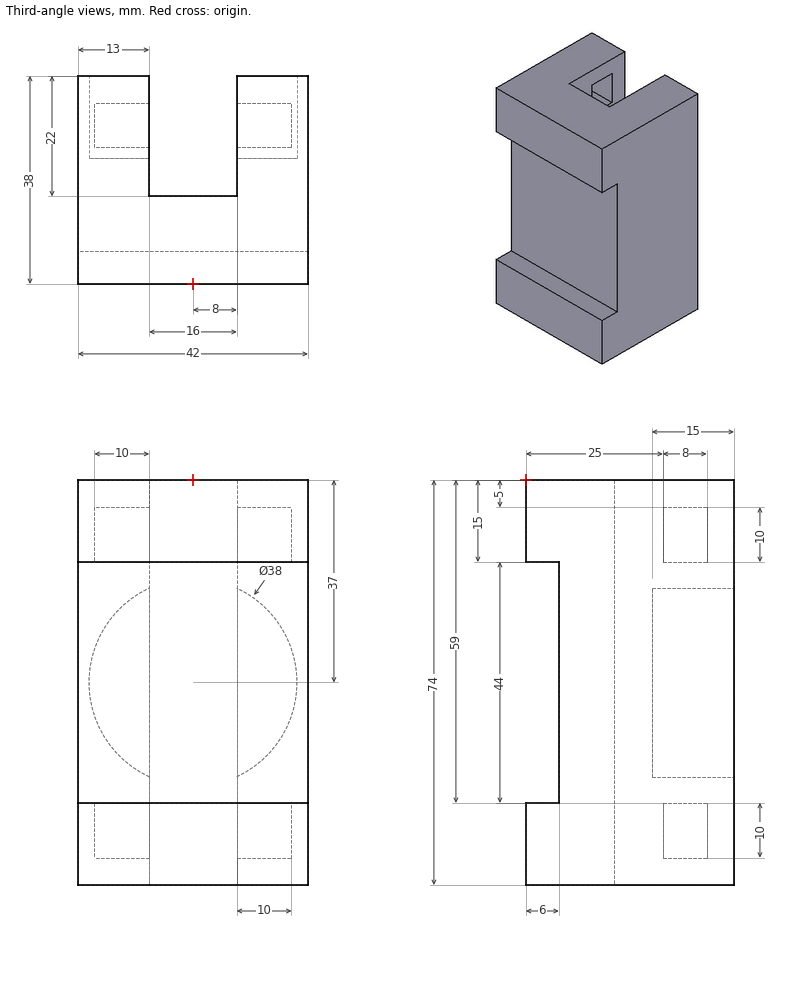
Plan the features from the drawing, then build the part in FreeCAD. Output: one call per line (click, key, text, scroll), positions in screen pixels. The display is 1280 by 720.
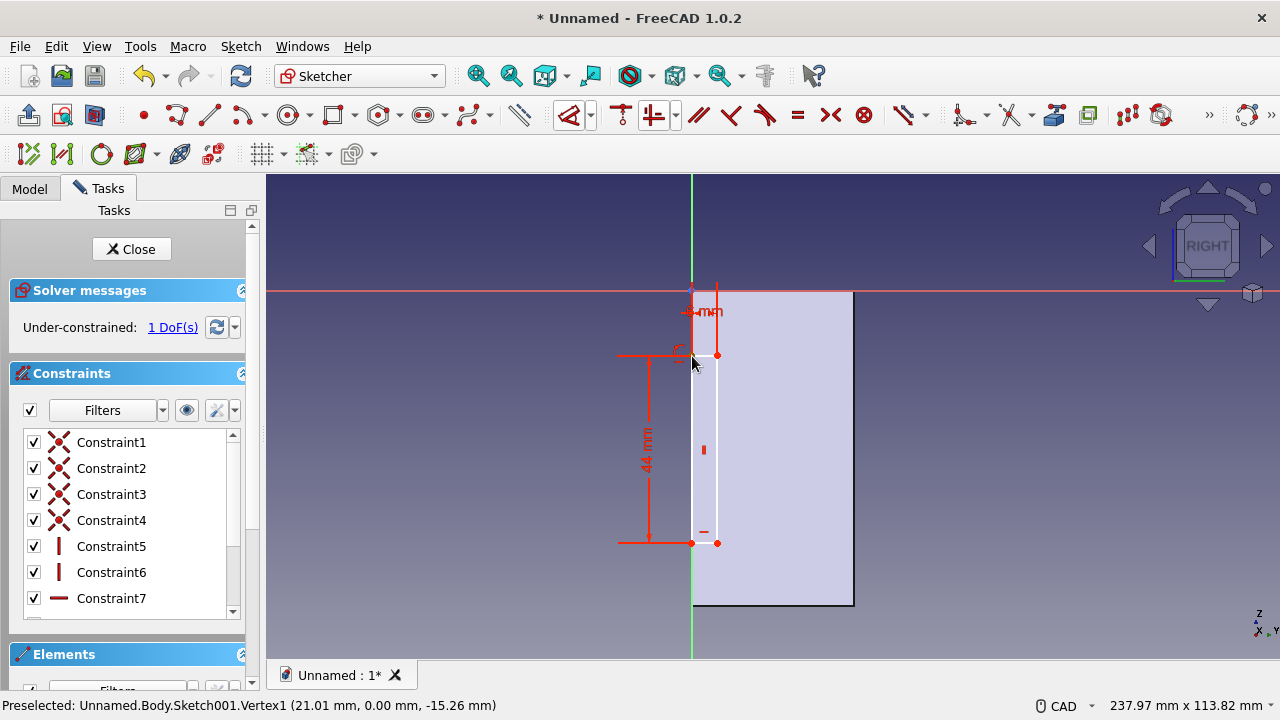
key(i)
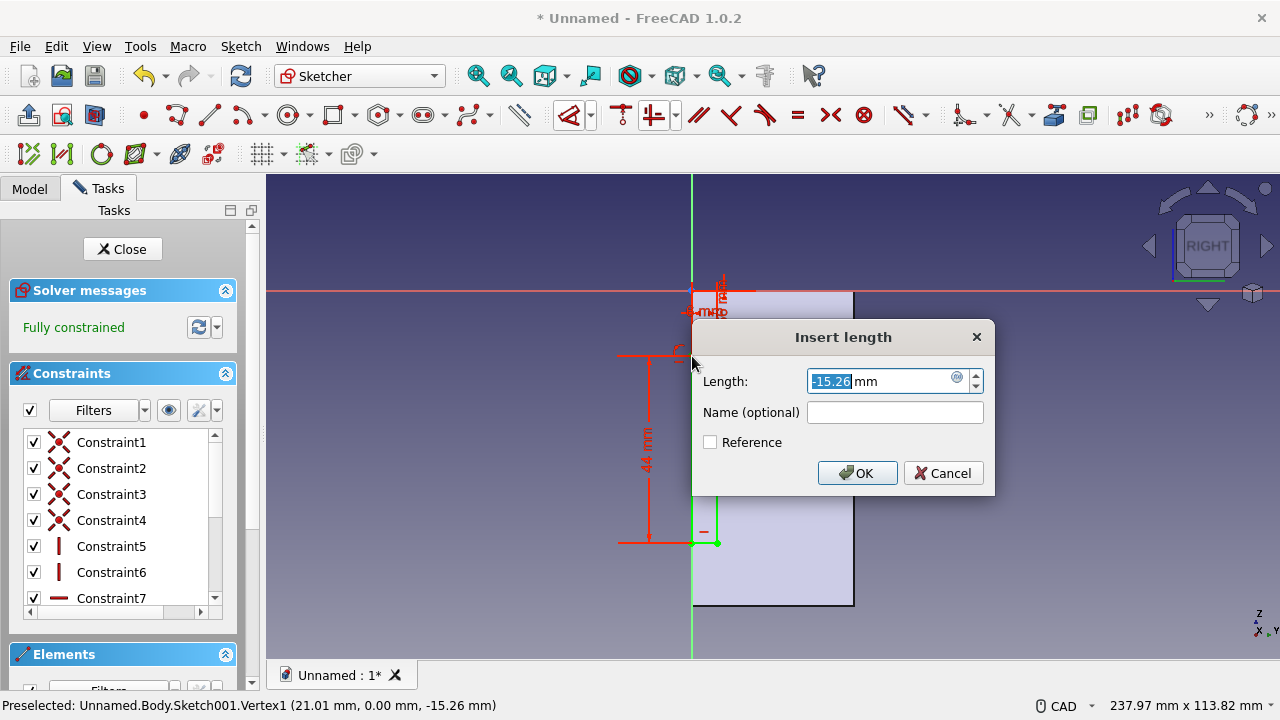
text(-15)
key(Return)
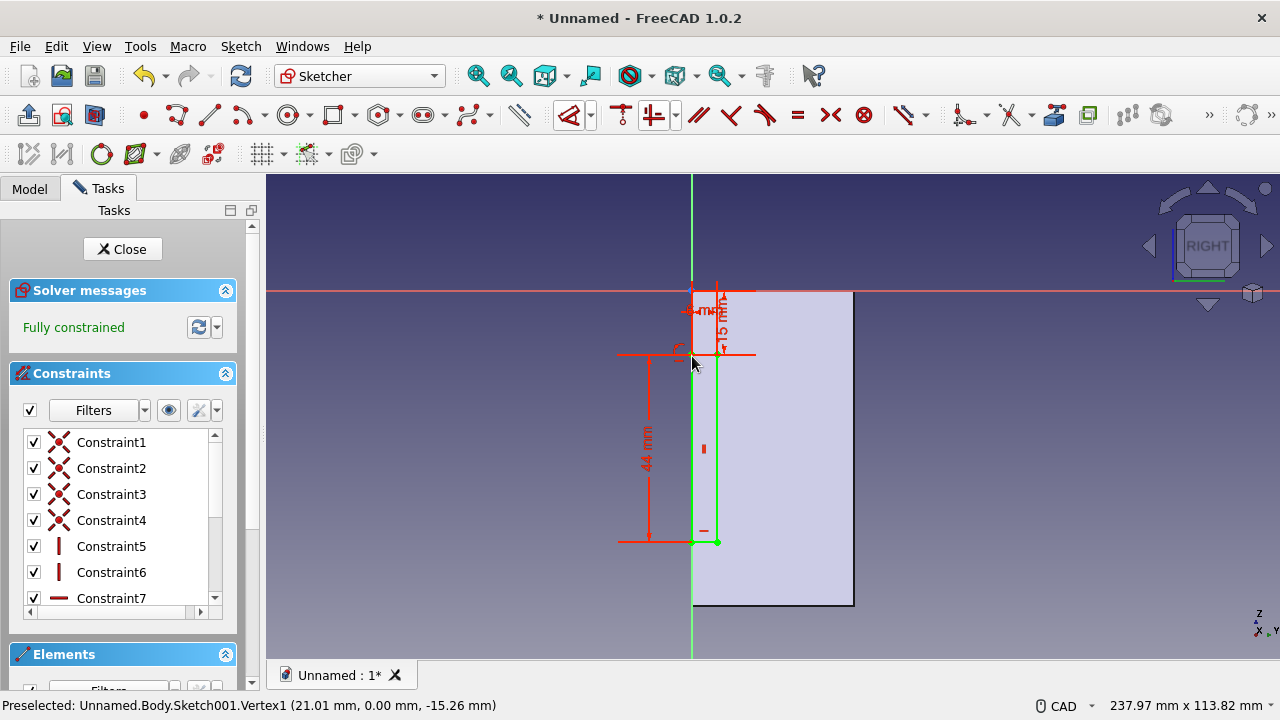
click(123, 249)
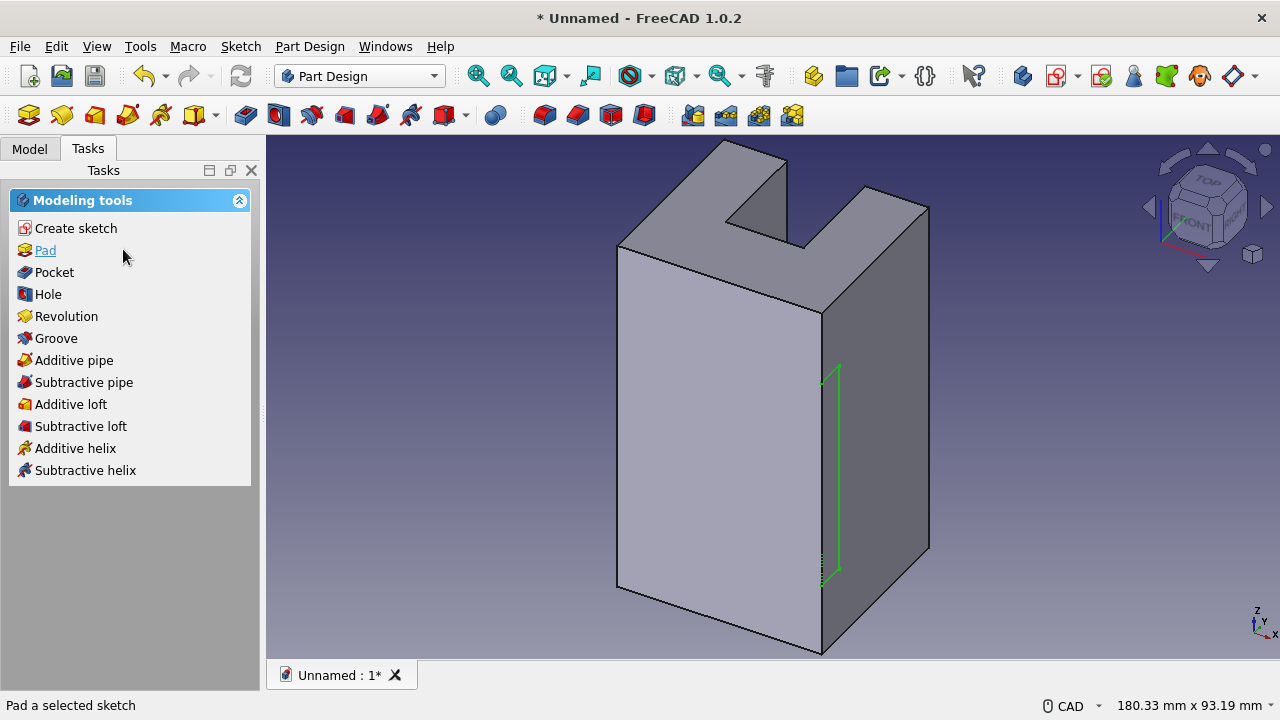
click(246, 116)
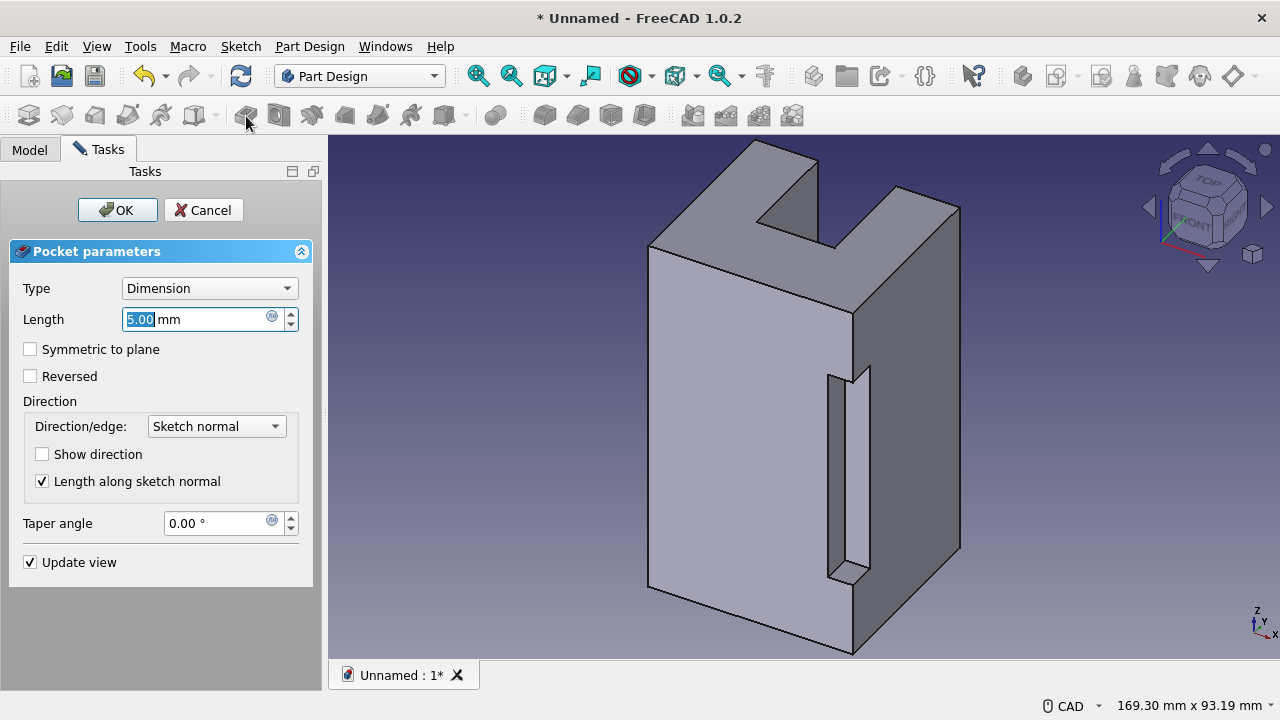
click(210, 288)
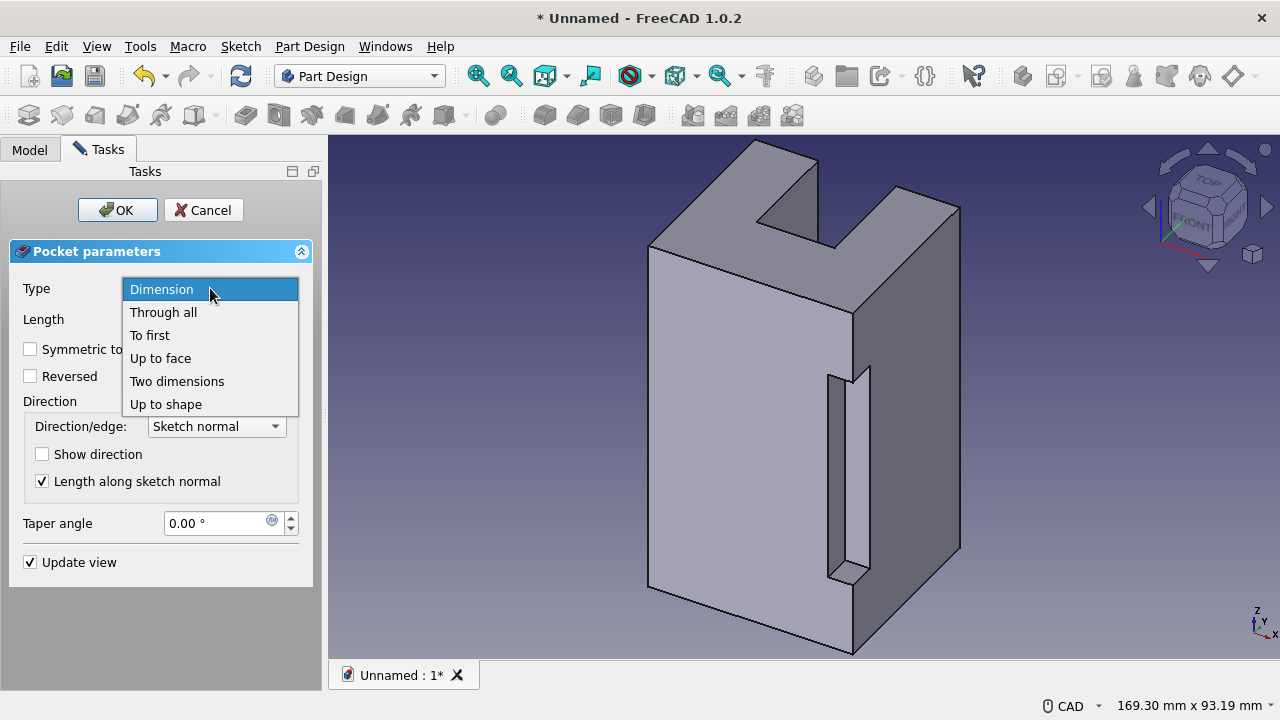
click(208, 312)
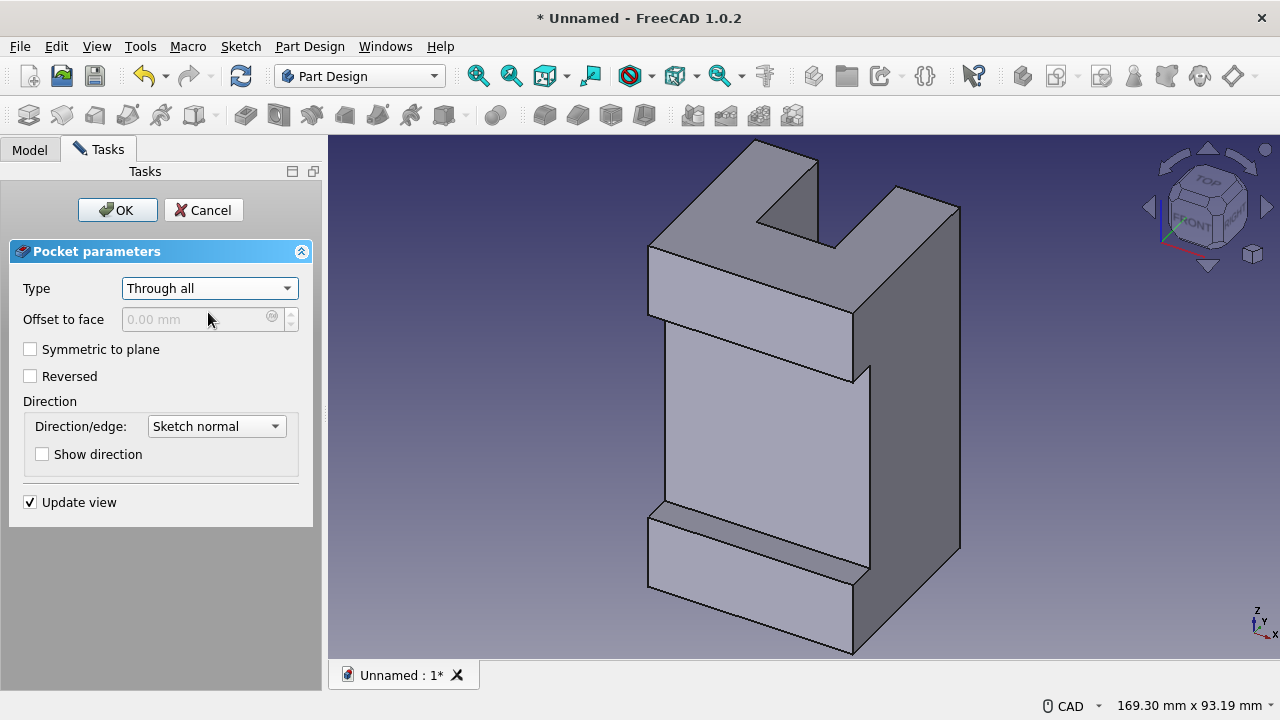
click(118, 210)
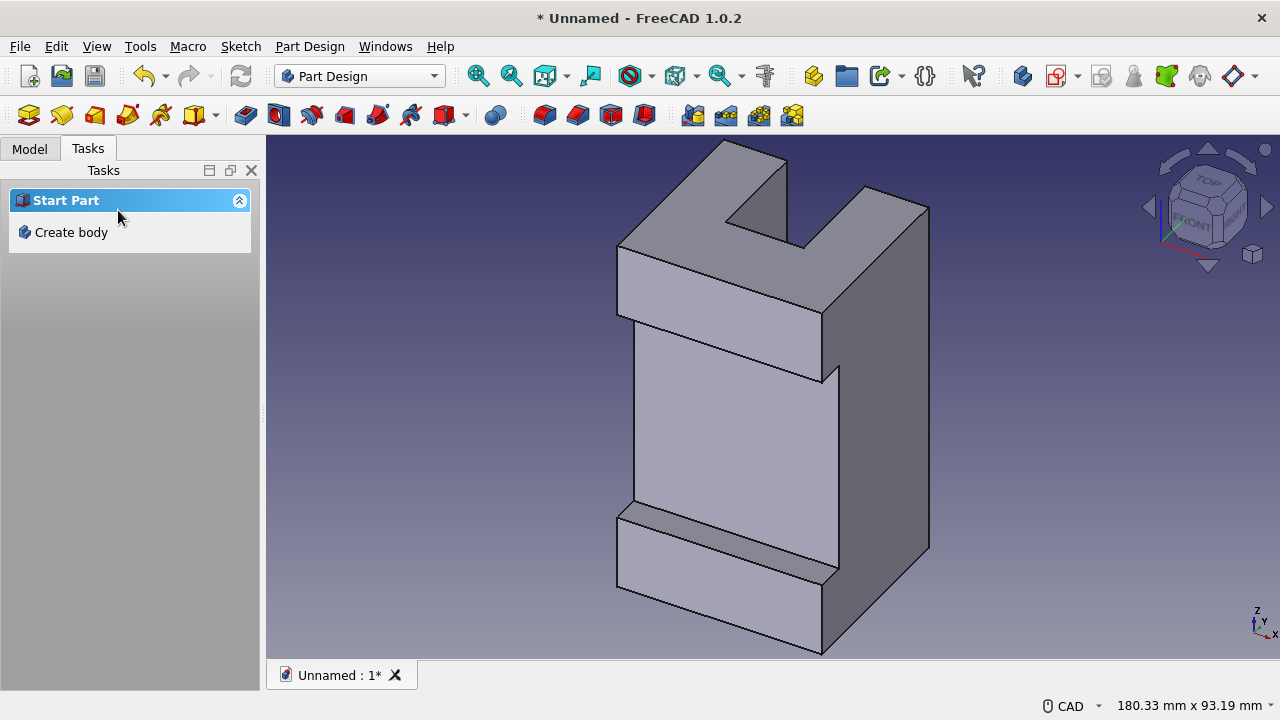
key(4)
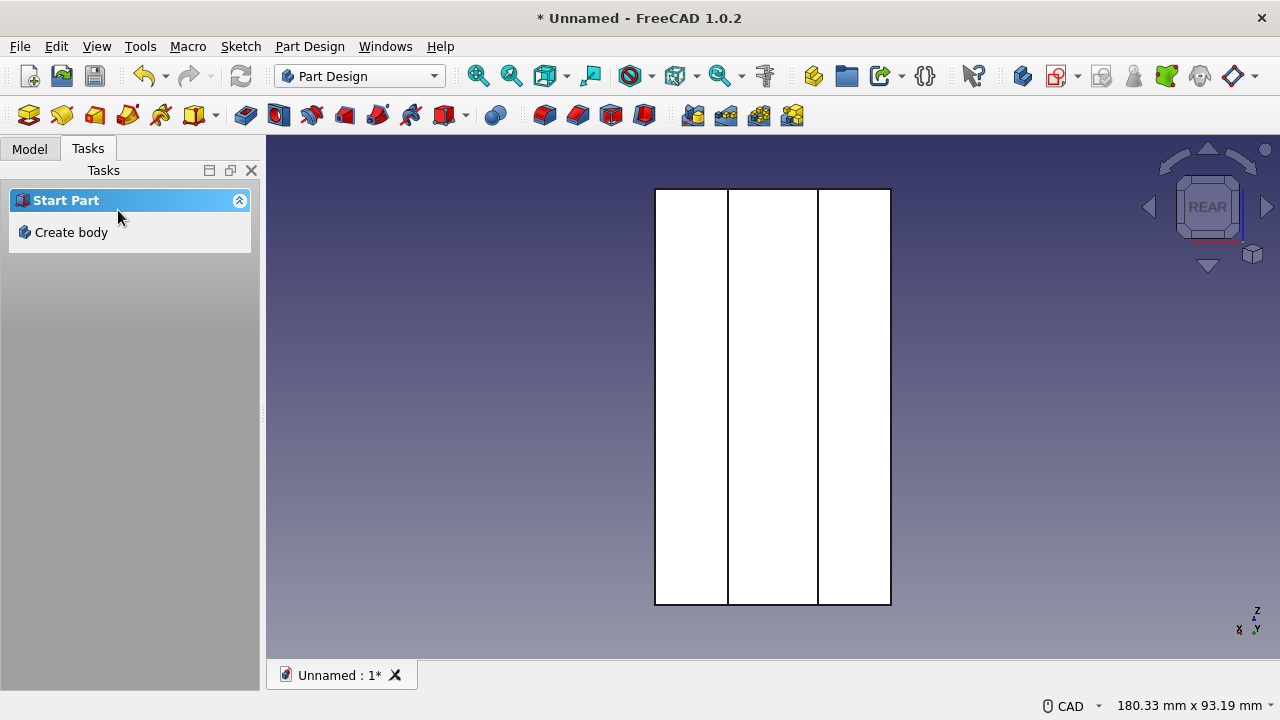
click(855, 277)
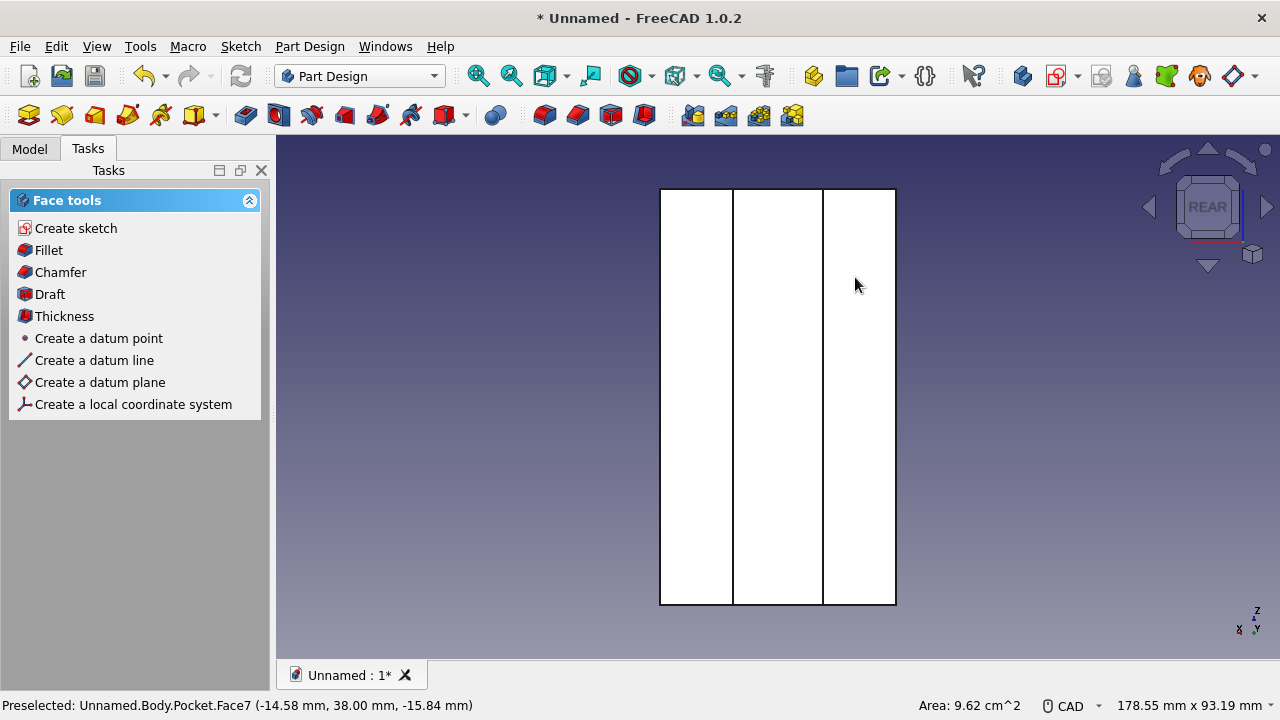
click(1056, 76)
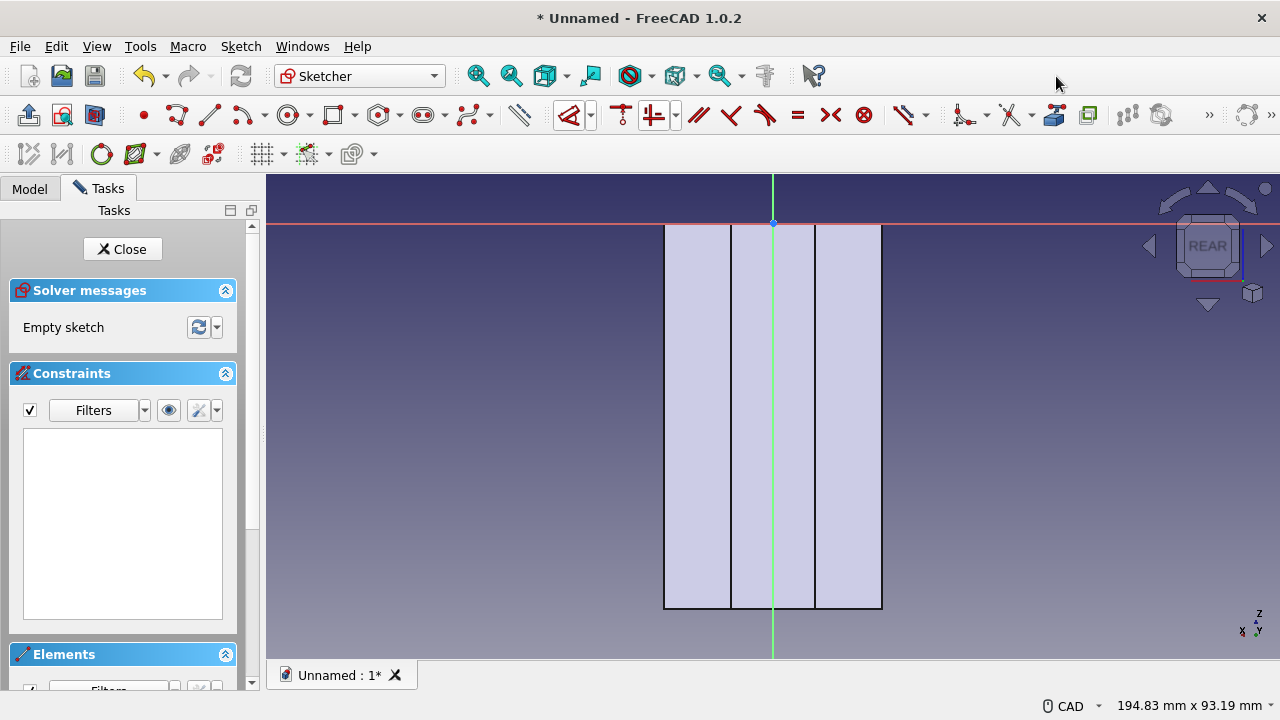
scroll(395, 628, down, 1)